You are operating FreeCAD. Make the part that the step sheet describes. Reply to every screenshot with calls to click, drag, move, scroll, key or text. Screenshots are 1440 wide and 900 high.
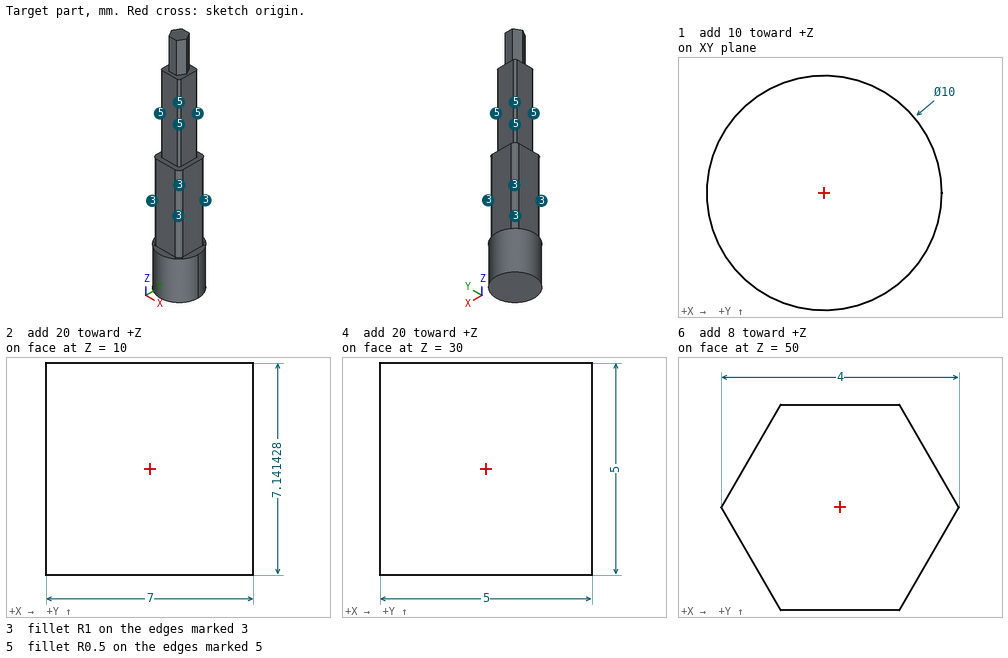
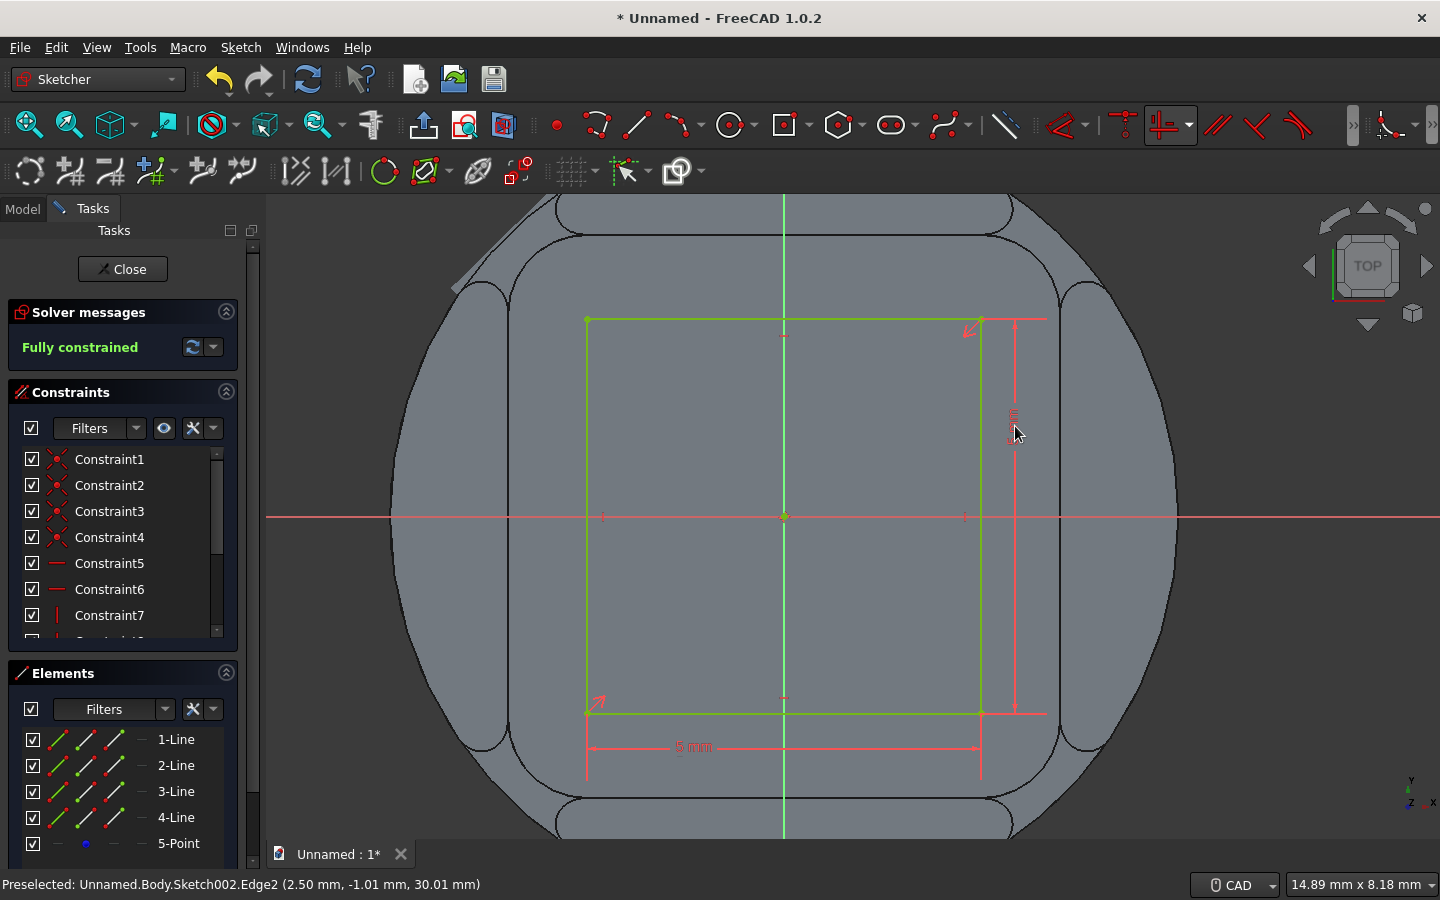
click(123, 269)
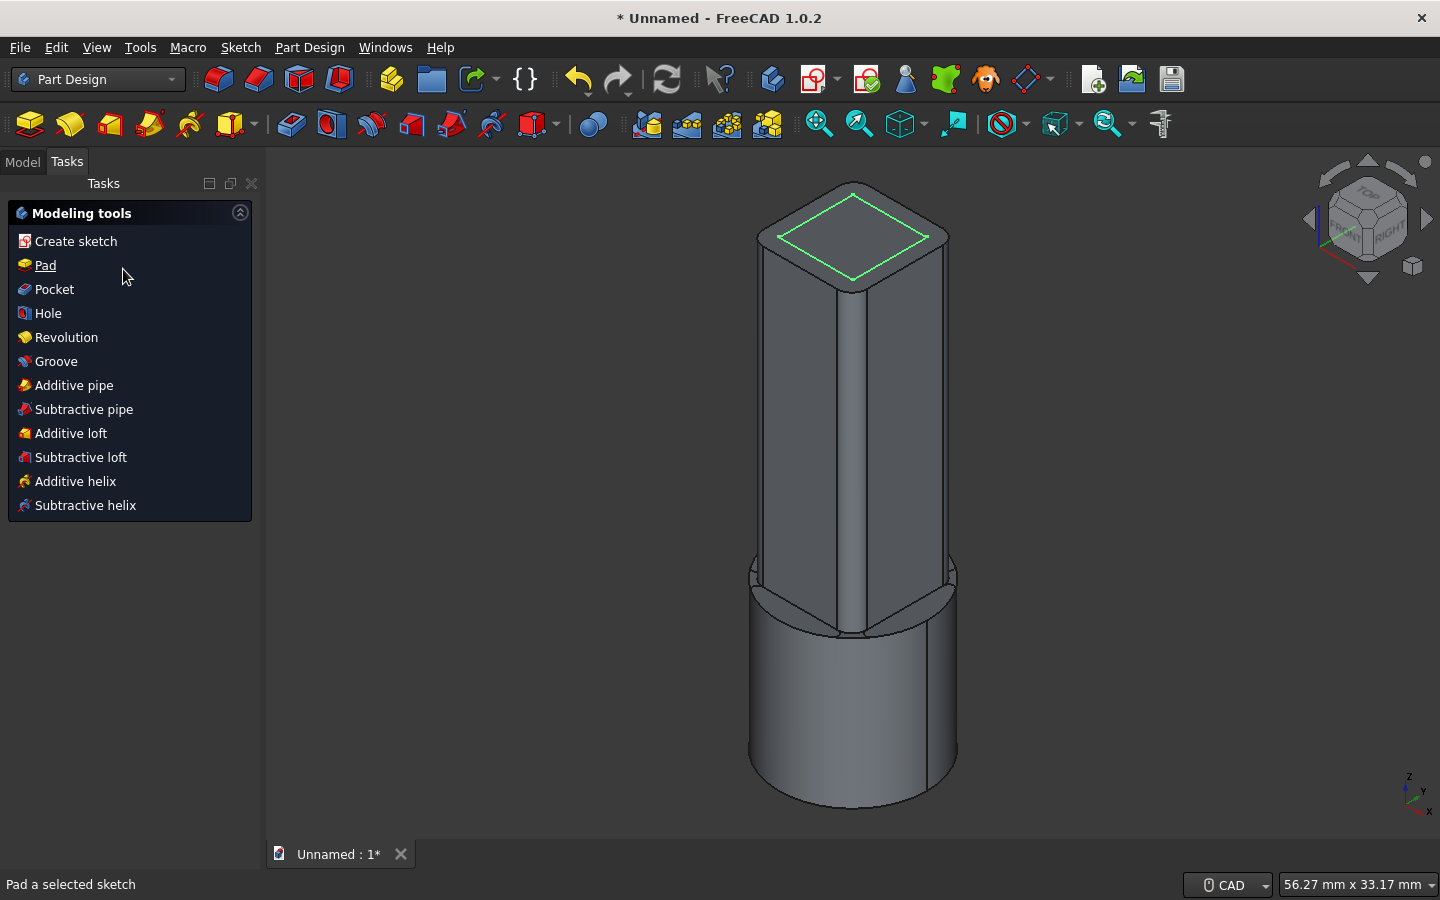
click(30, 124)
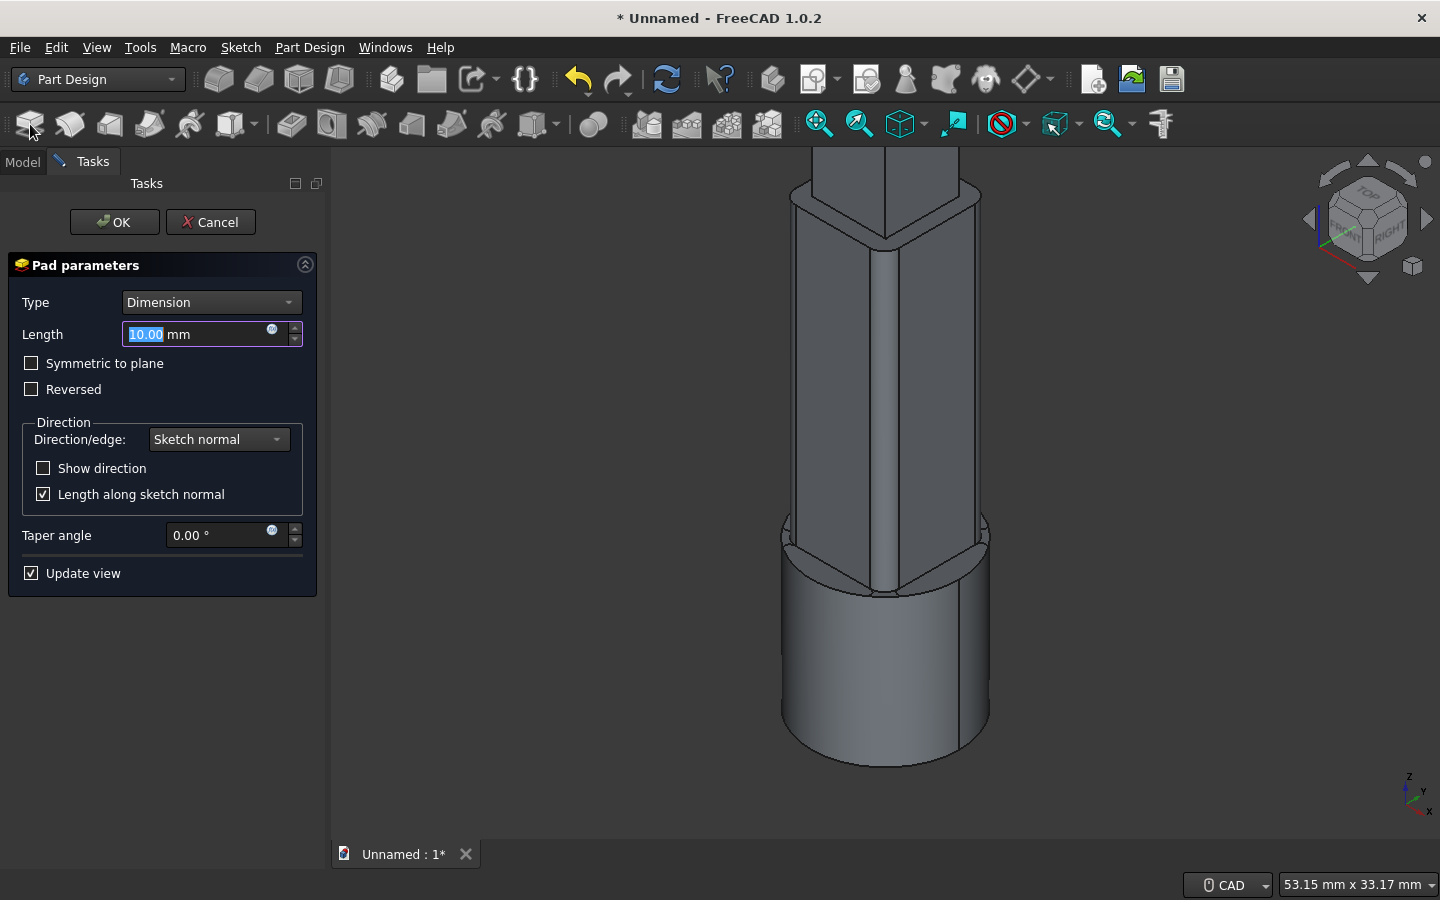
text(20)
key(Tab)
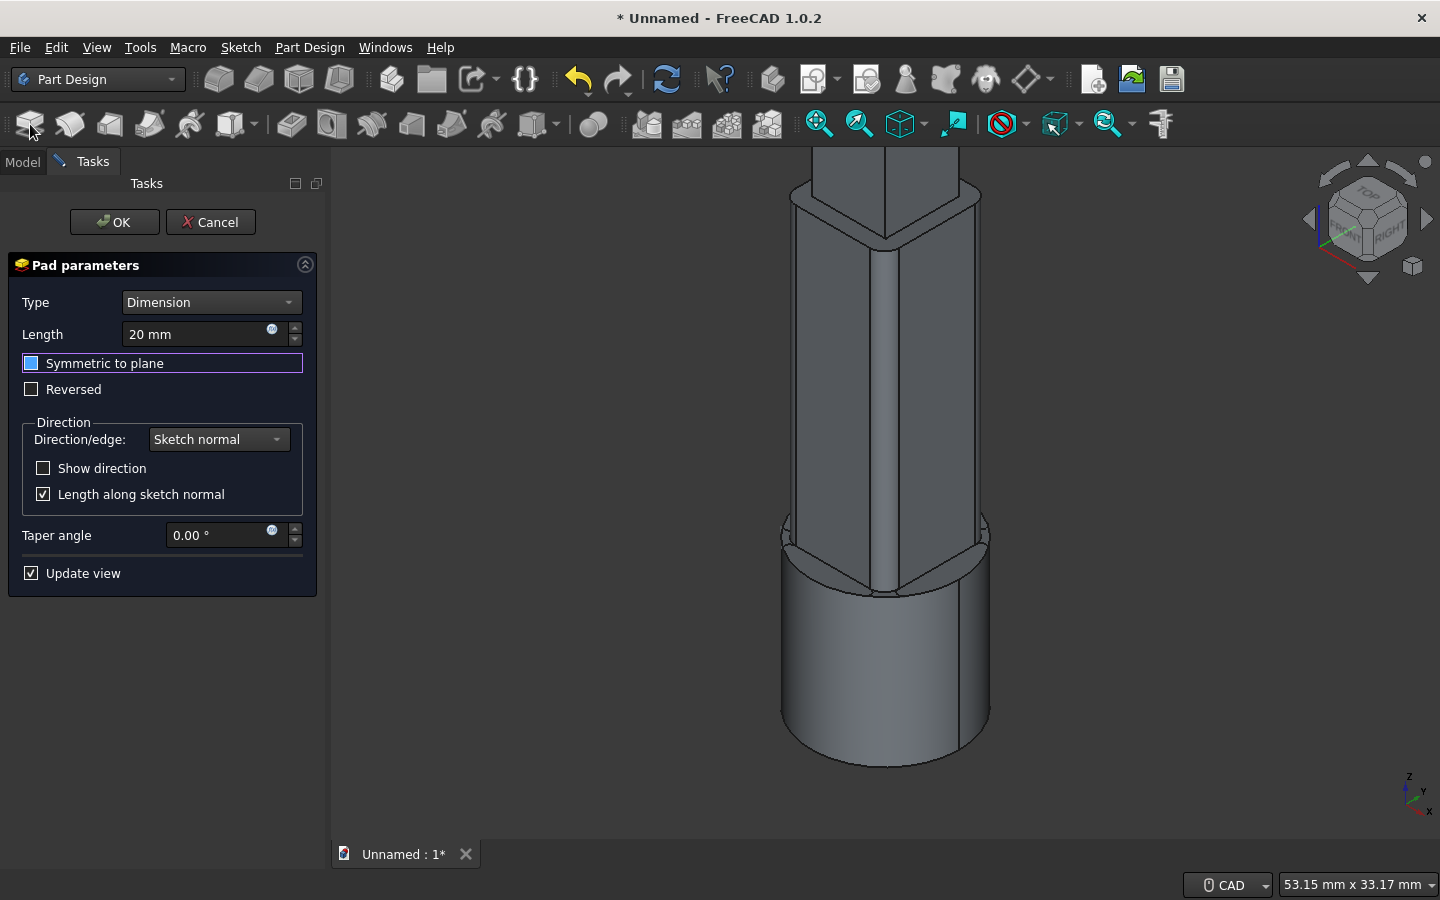
click(115, 222)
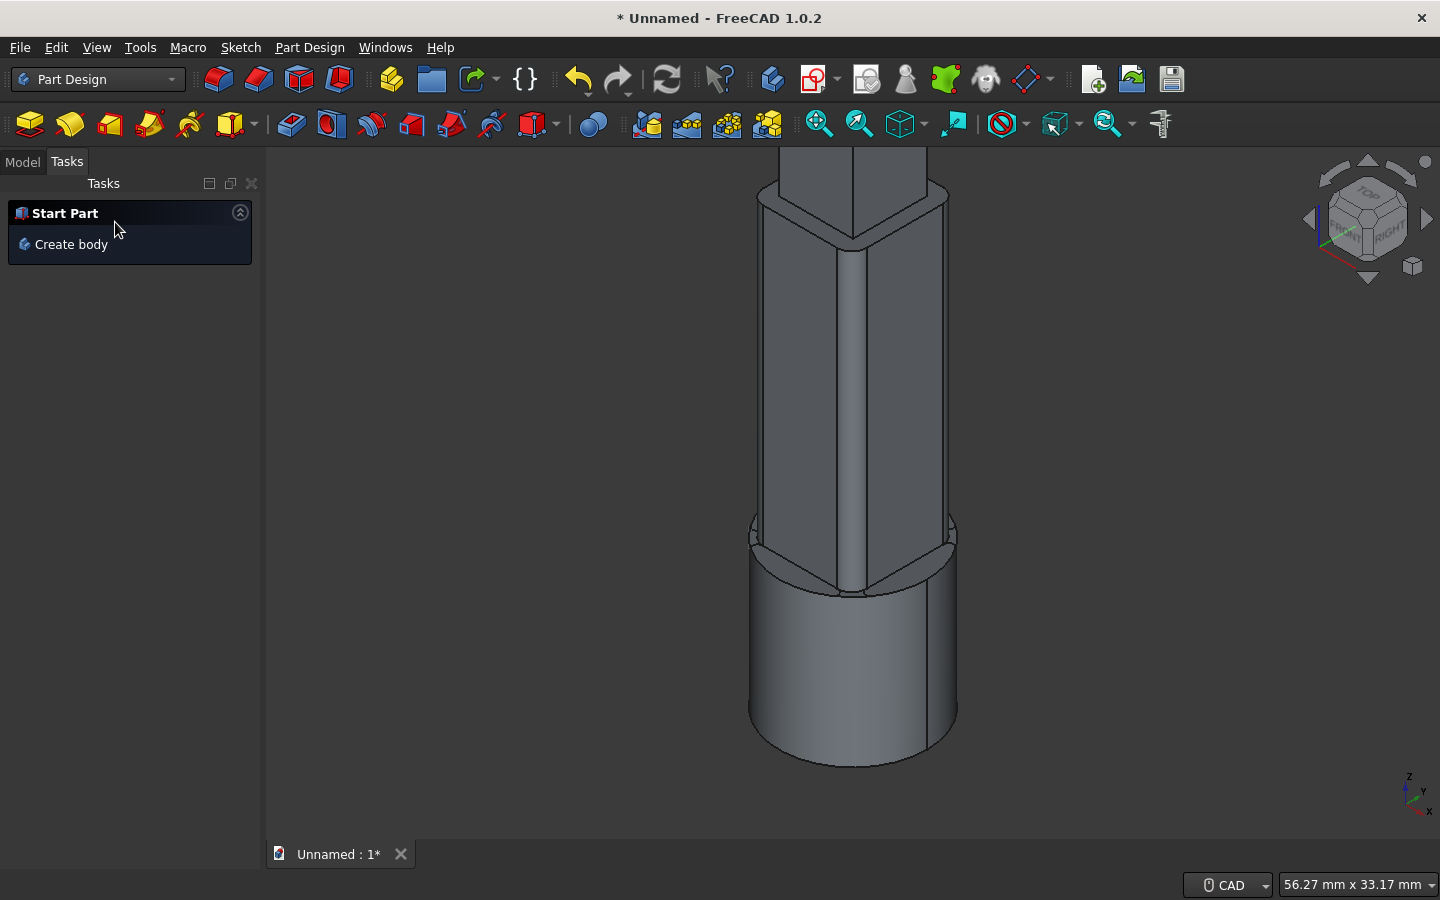
key(v)
key(f)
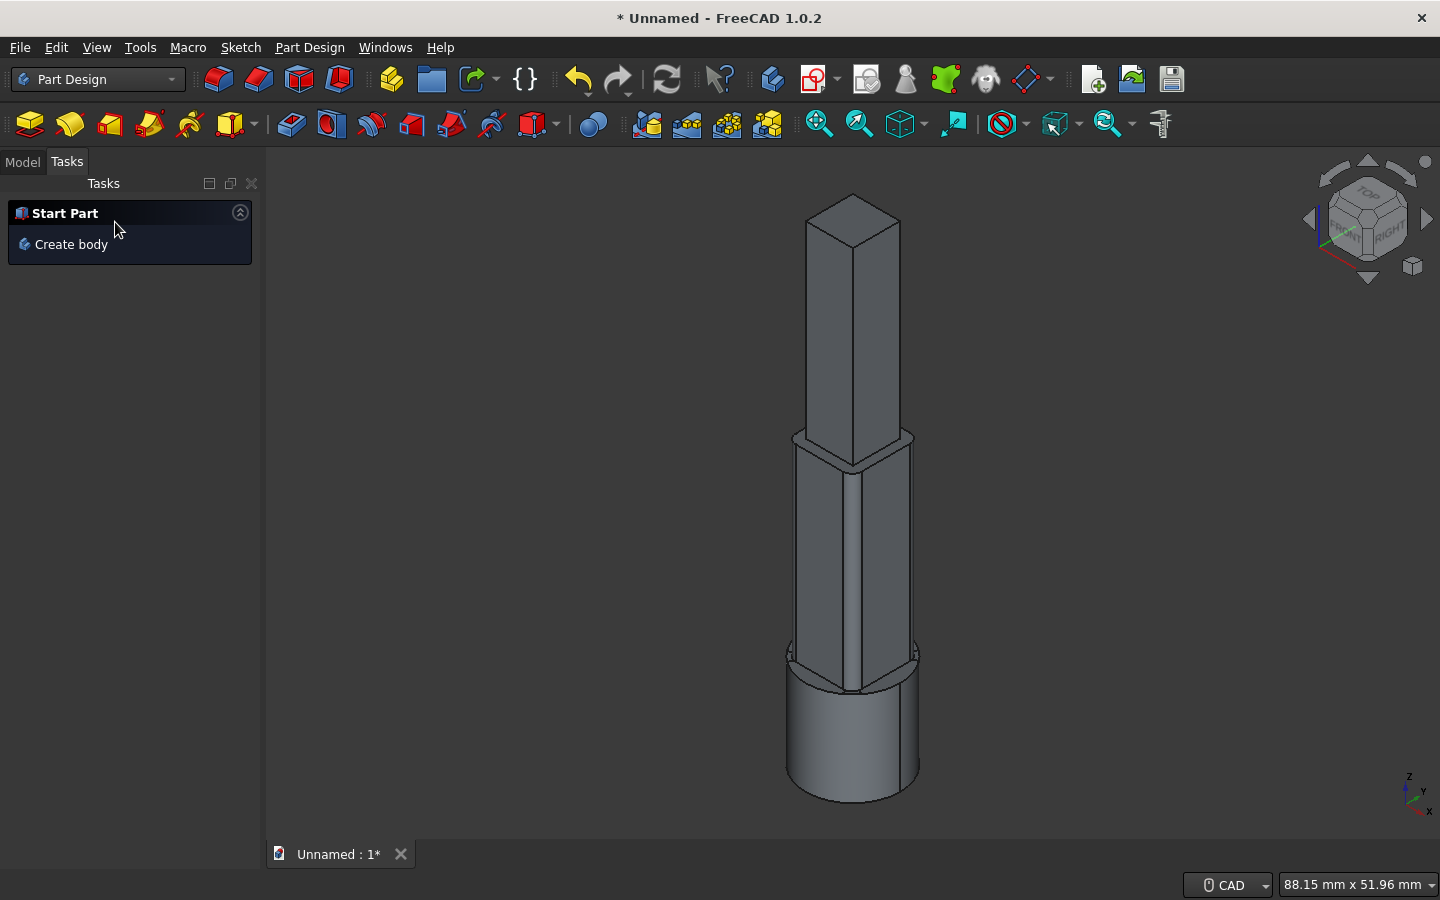
click(853, 356)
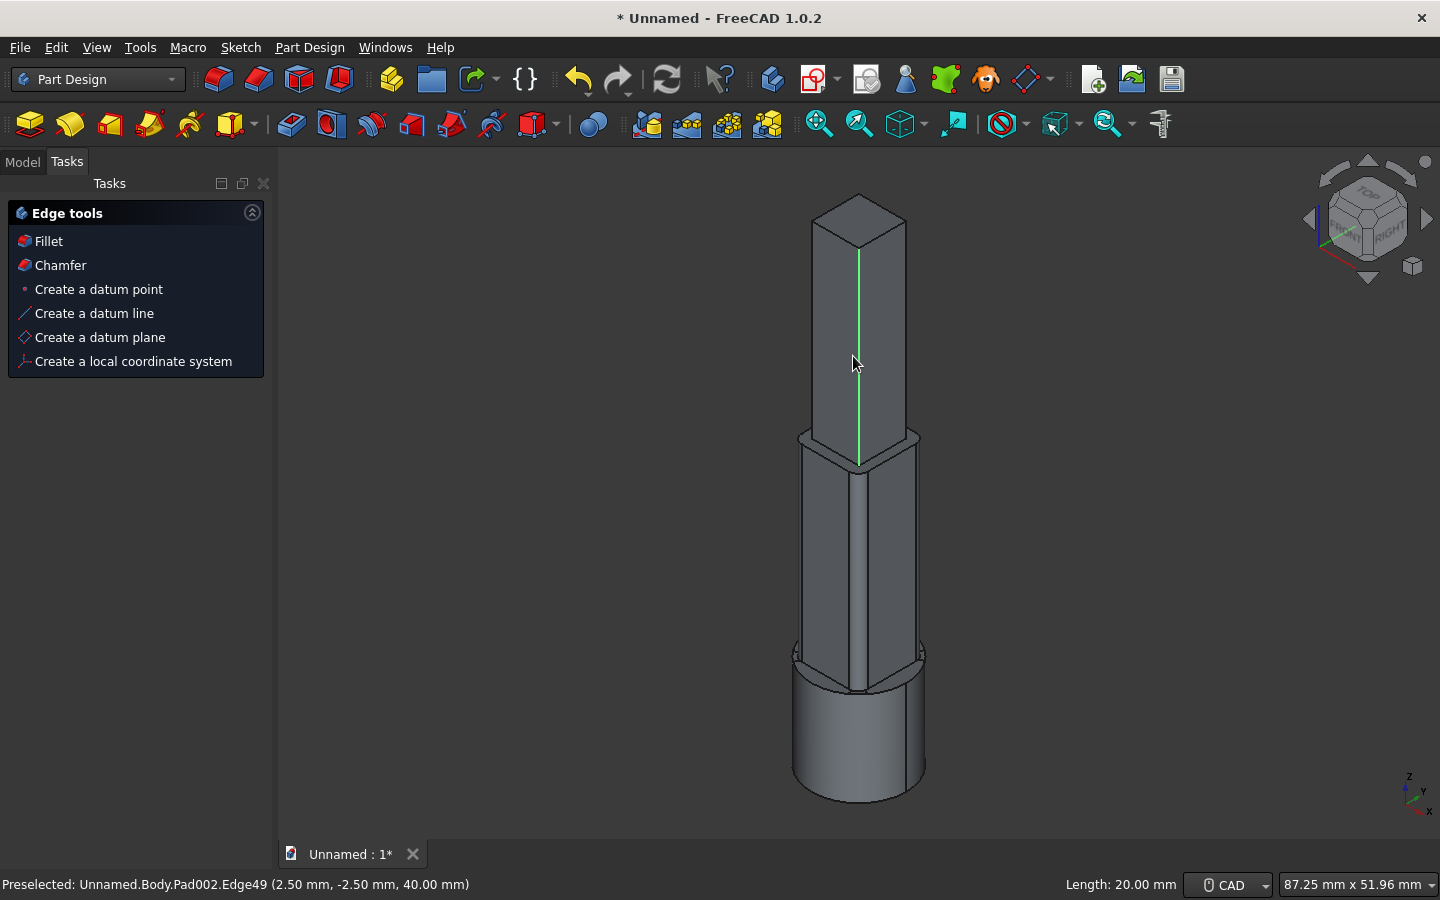
key(2)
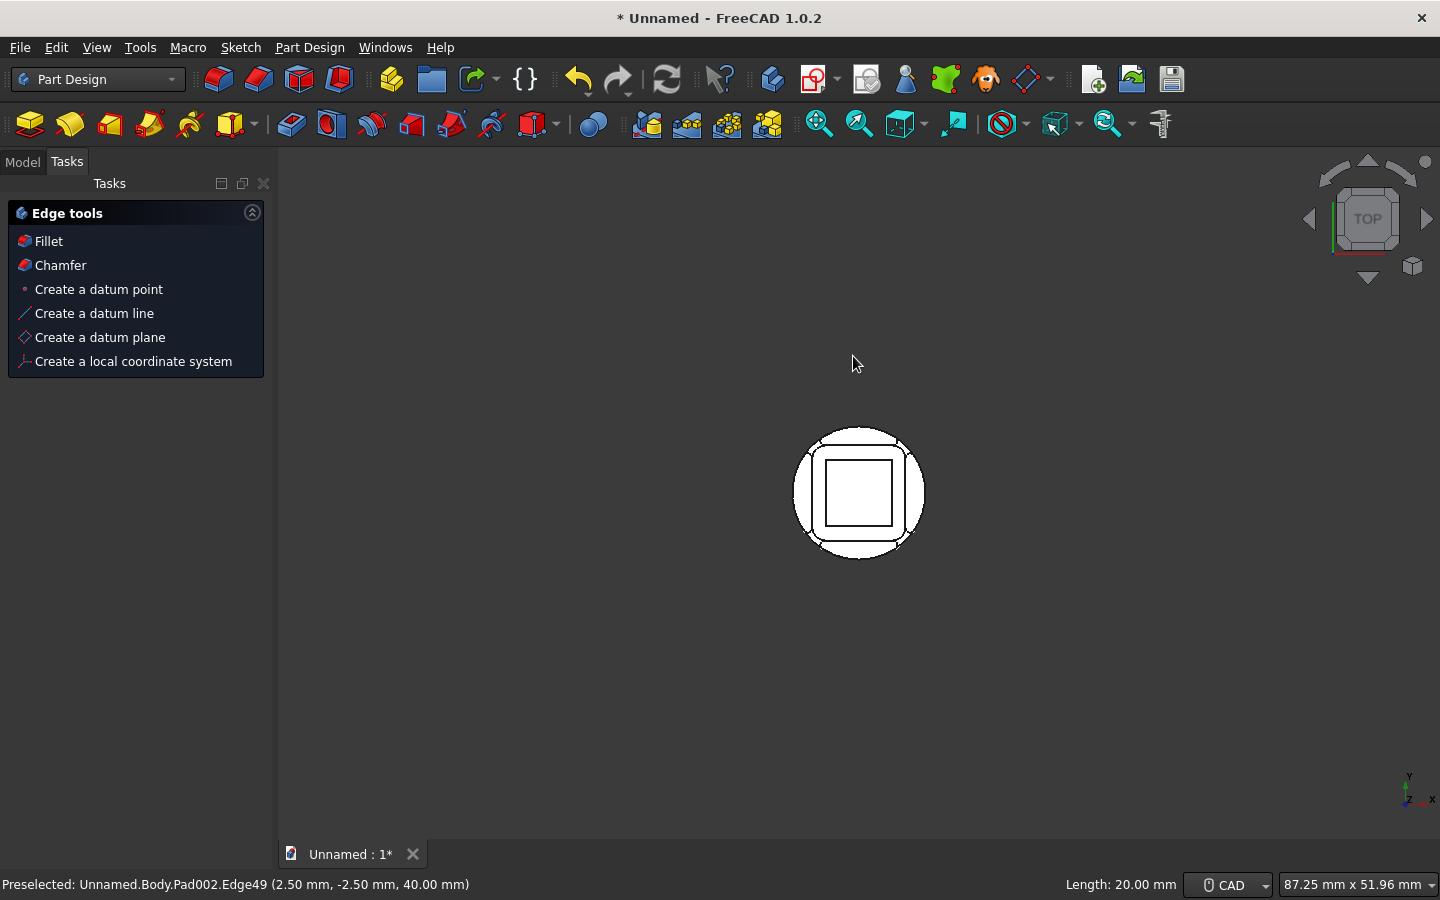
click(820, 124)